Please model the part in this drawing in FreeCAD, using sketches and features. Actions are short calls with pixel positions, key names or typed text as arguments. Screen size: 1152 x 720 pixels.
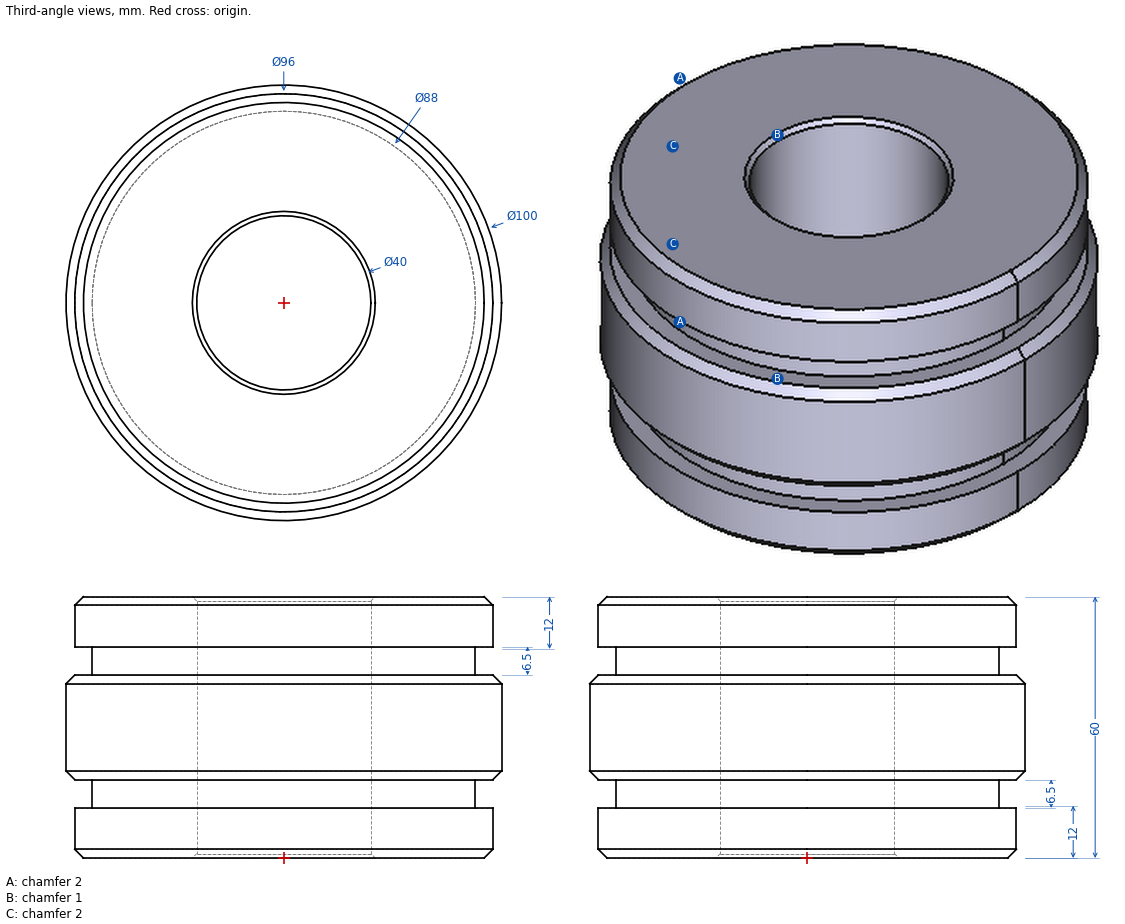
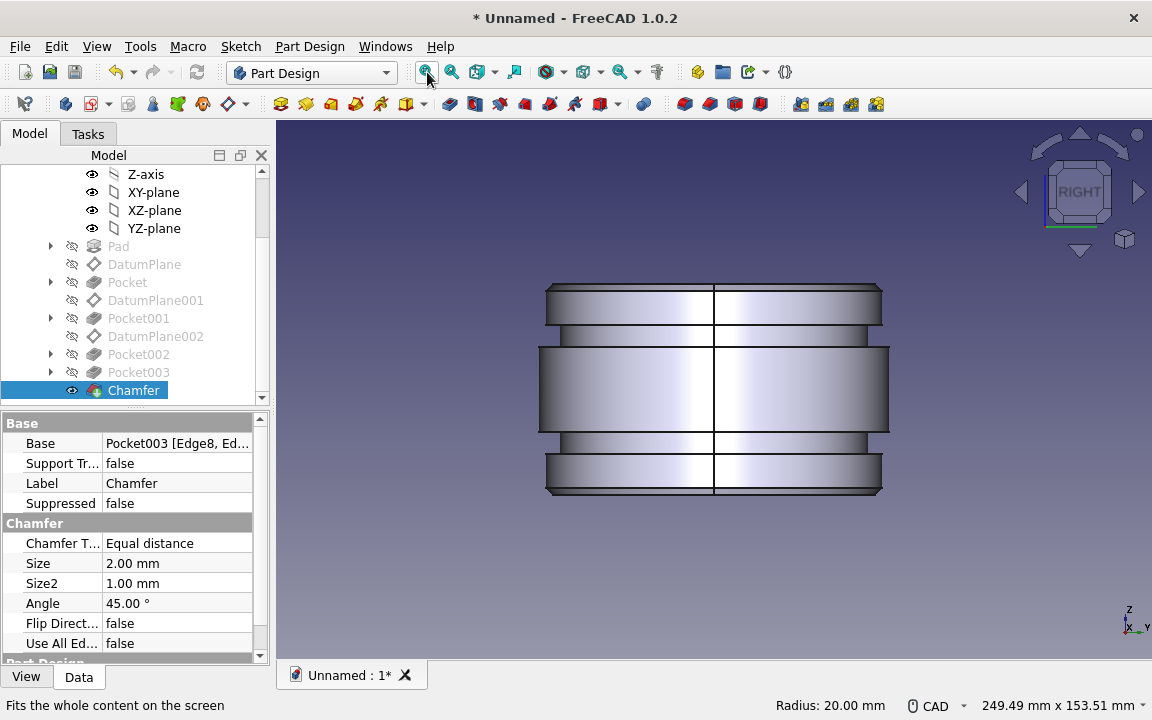
key(5)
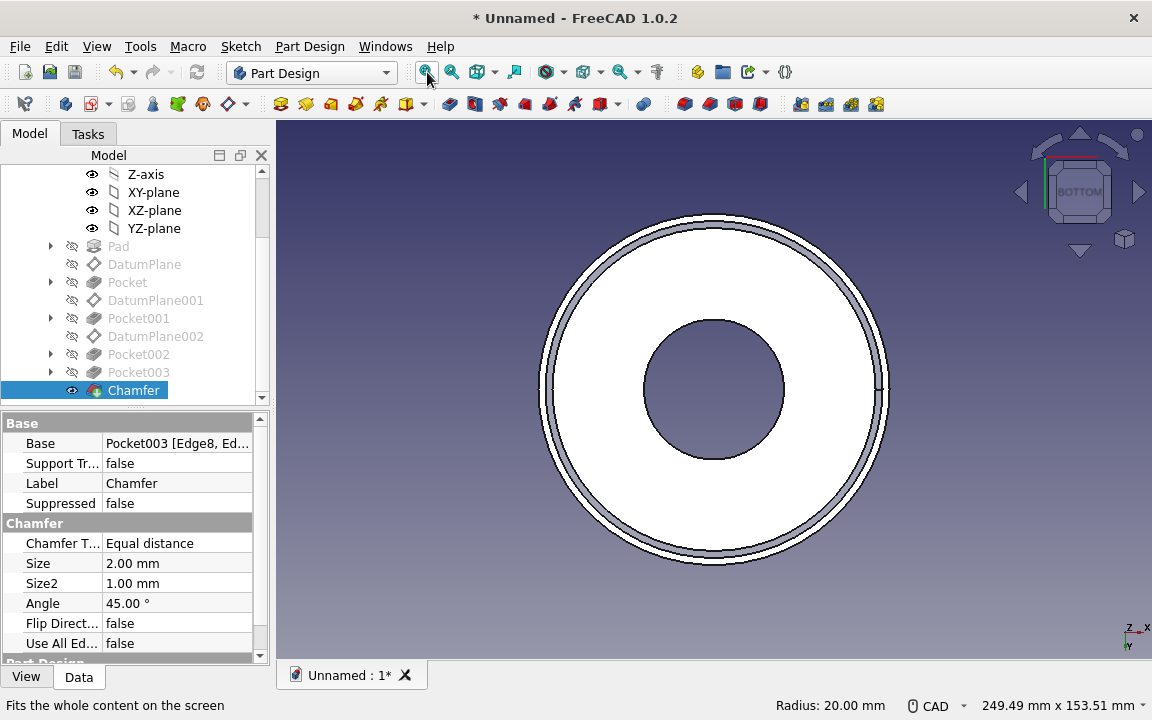
click(692, 455, ctrl)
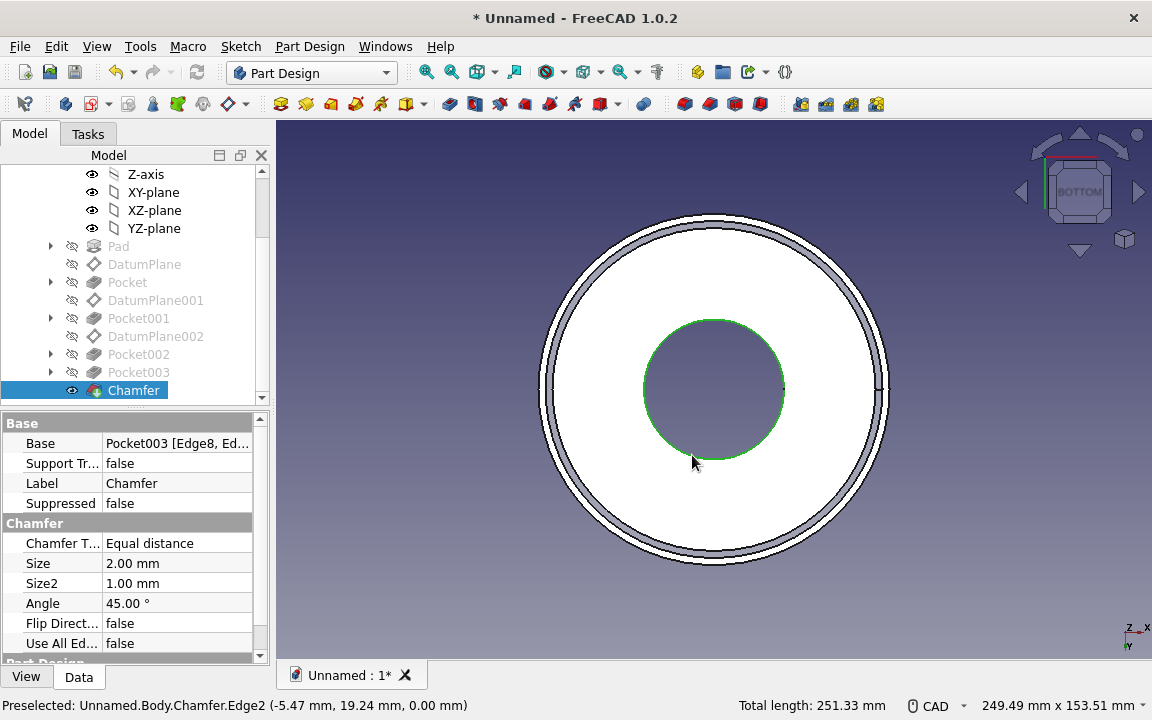
click(710, 104)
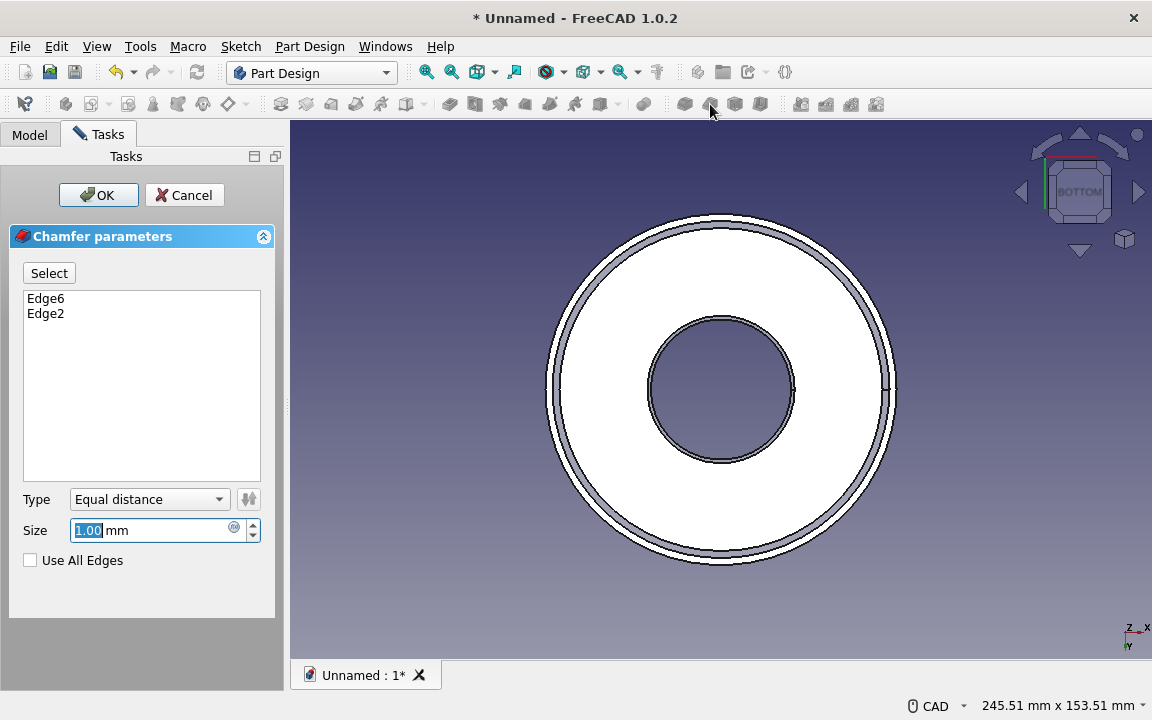
text(1)
key(Tab)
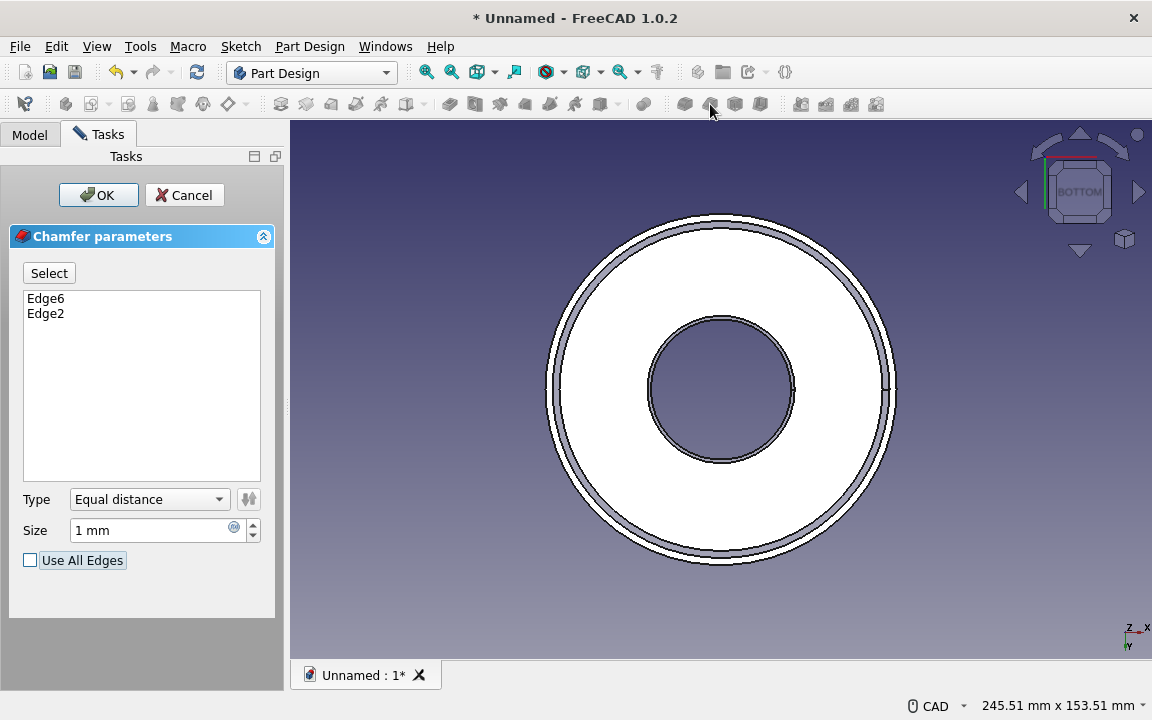
click(99, 195)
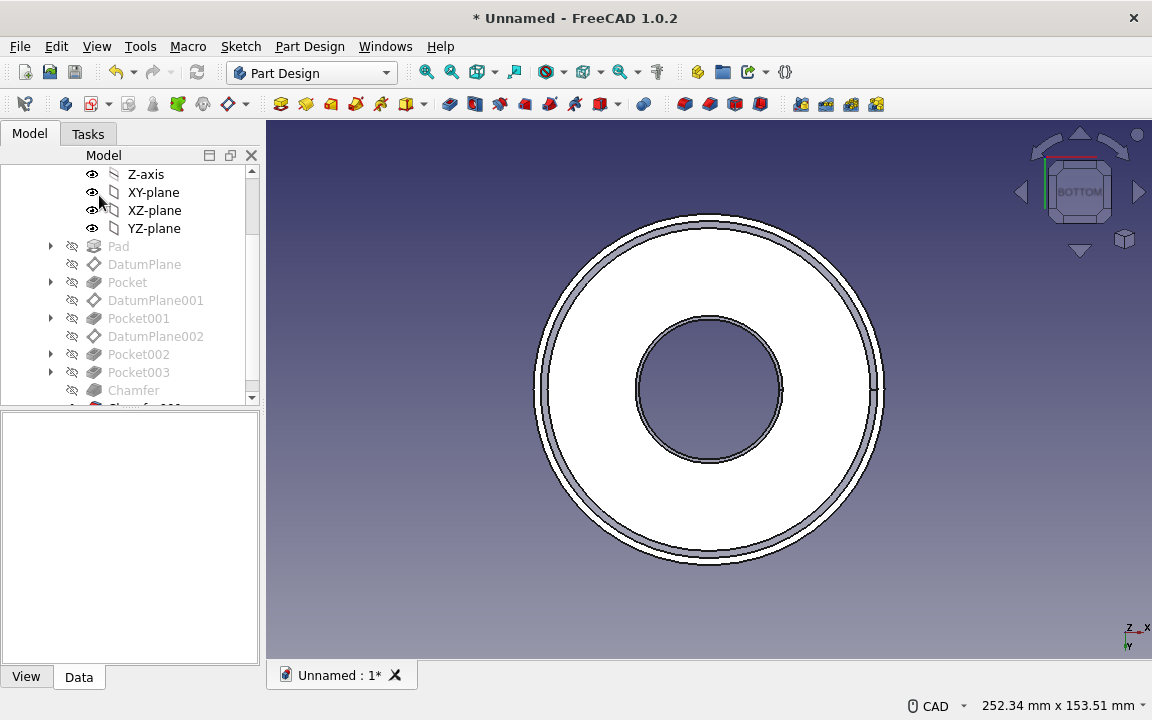
click(533, 388)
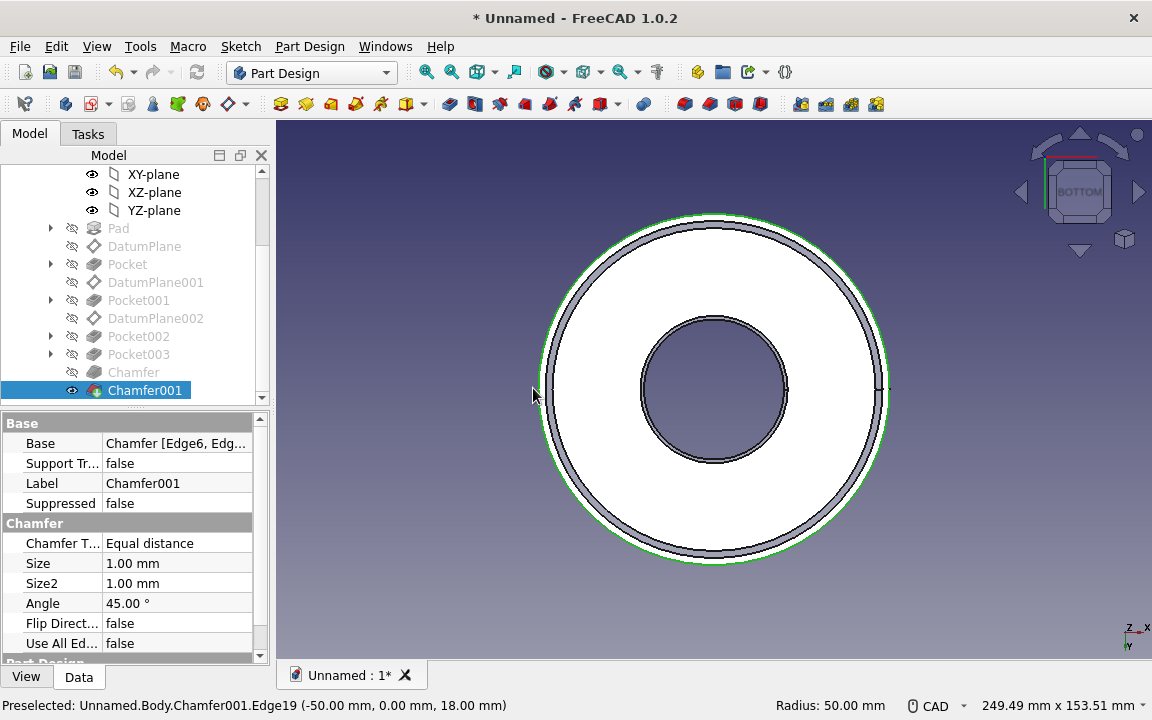
key(0)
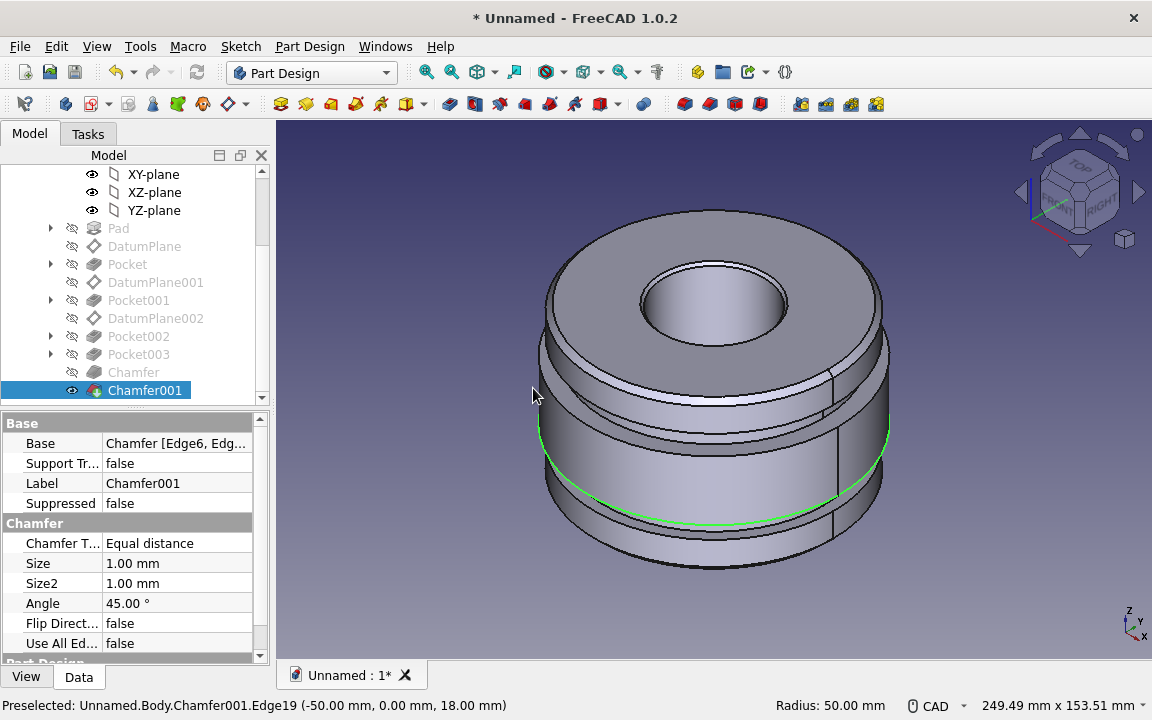
click(558, 400, ctrl)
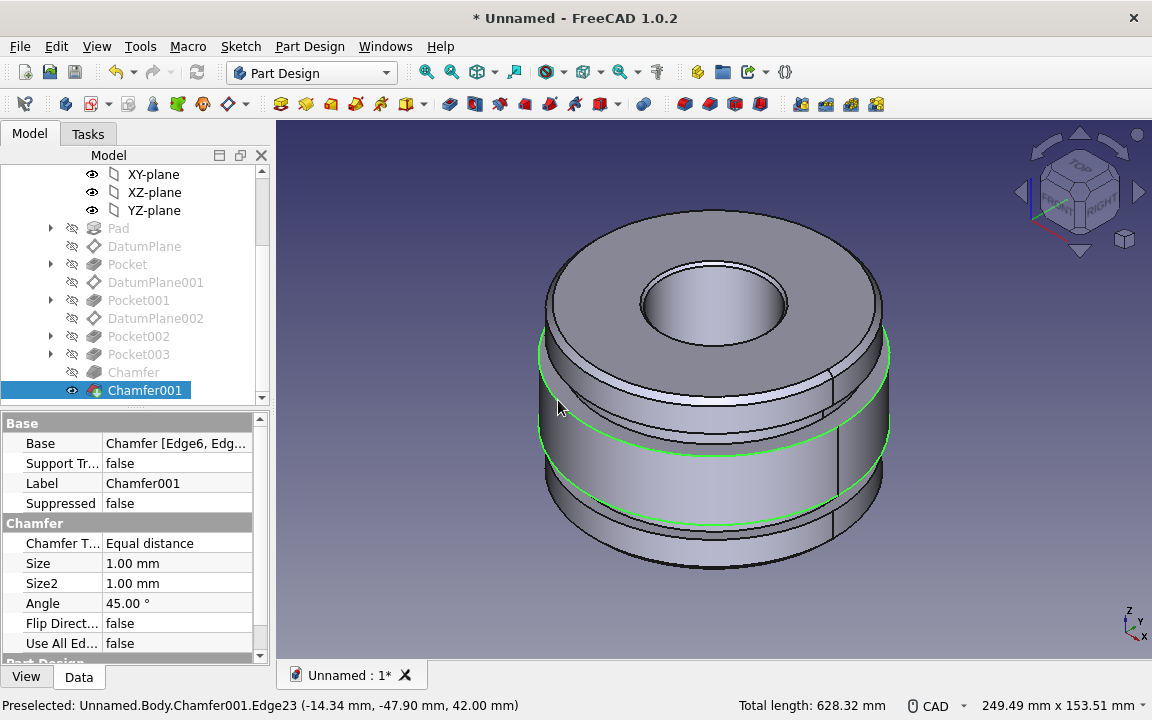
click(710, 104)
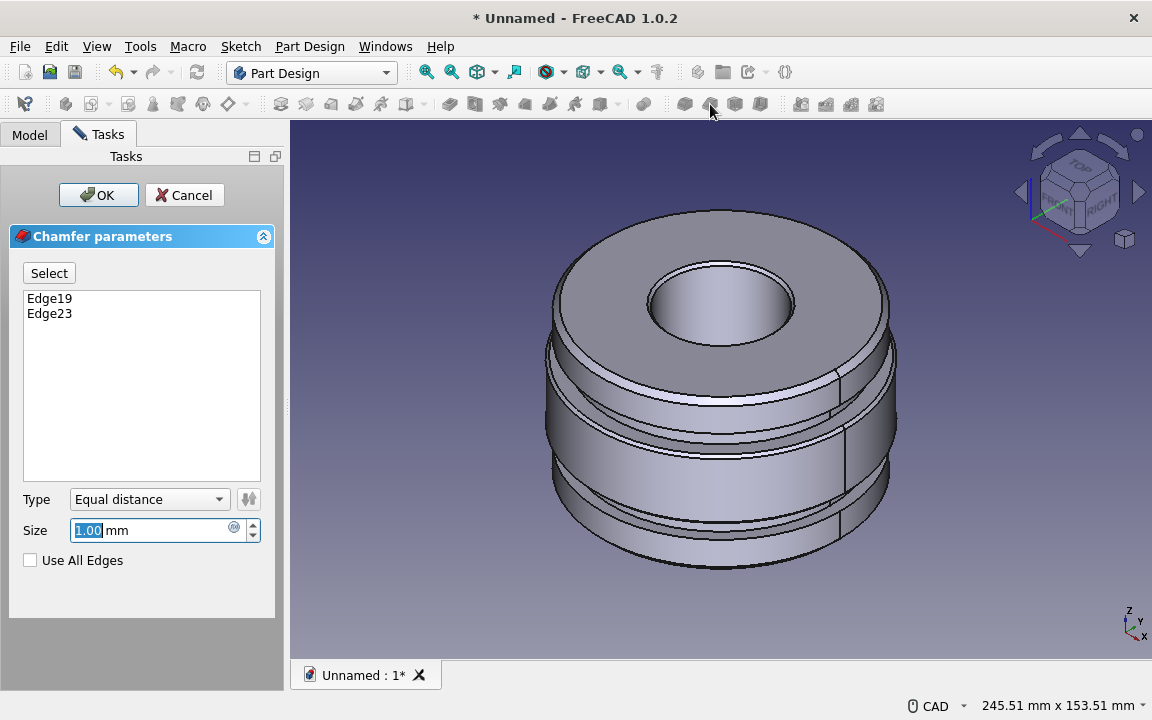
text(2)
key(Tab)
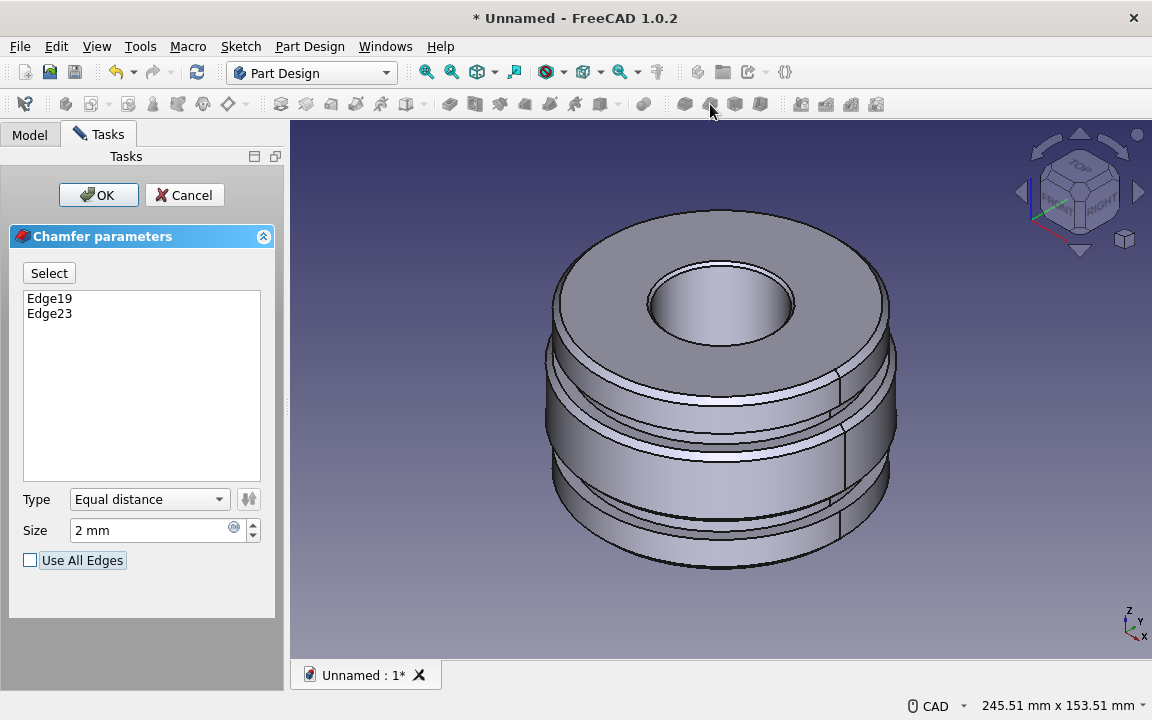
click(99, 195)